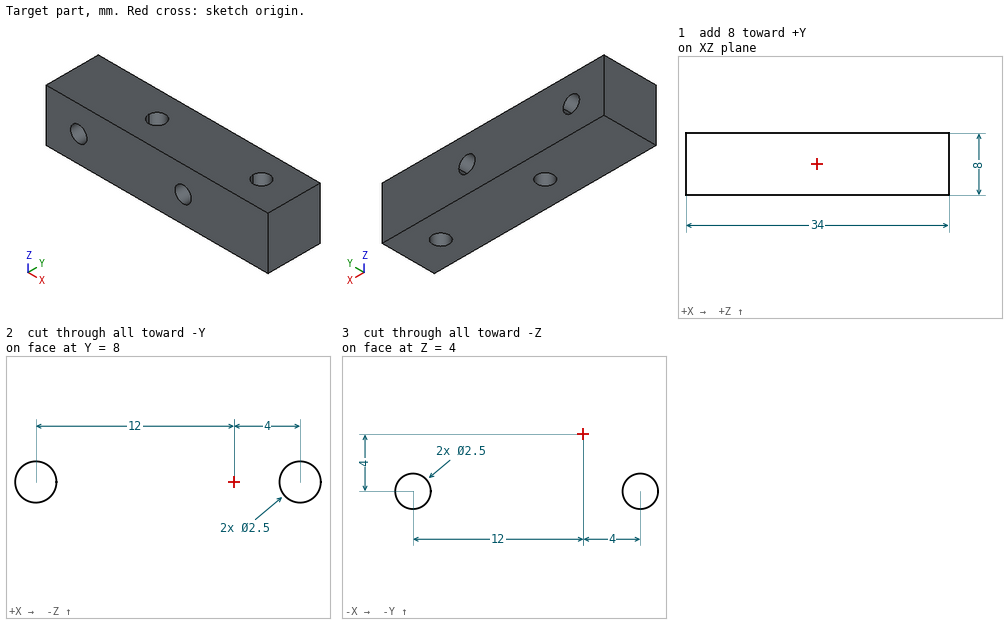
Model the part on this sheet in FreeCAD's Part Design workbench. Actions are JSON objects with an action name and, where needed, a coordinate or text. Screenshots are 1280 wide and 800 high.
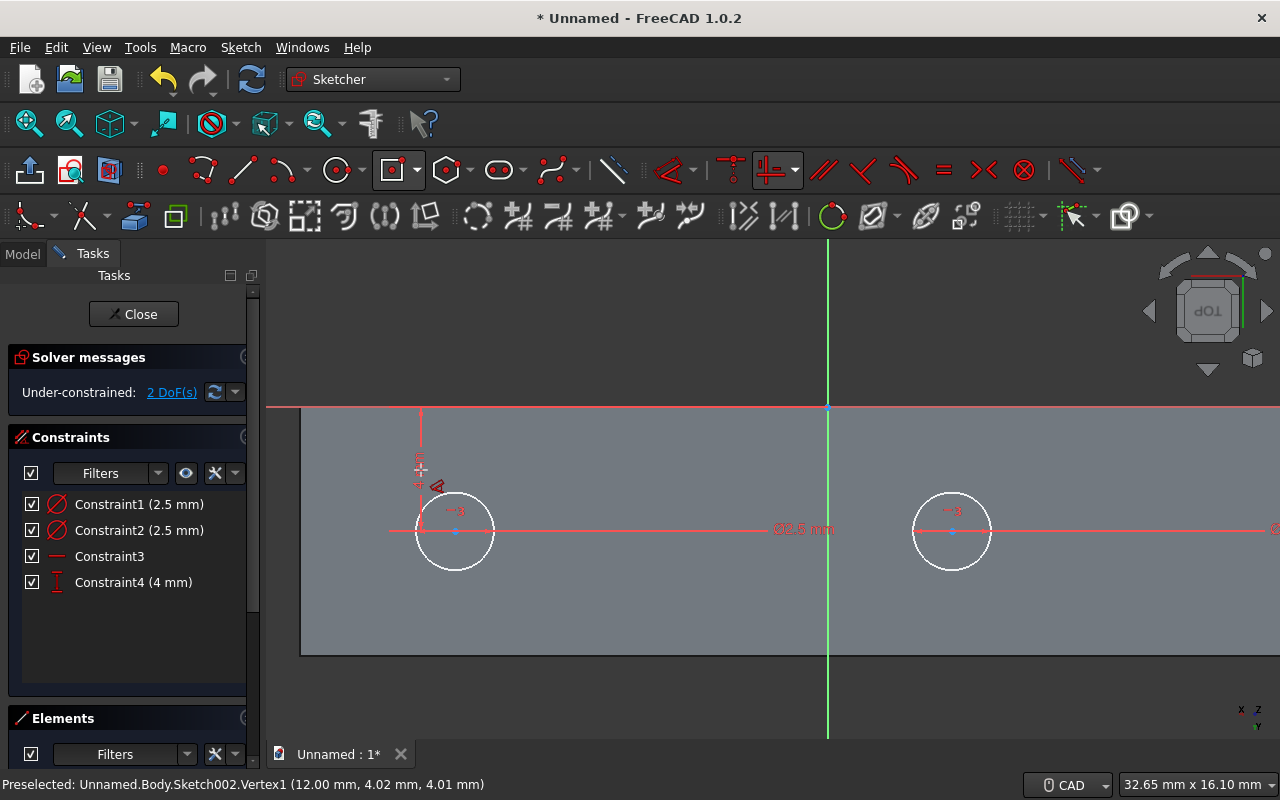
{"action": "left_click", "coordinate": [952, 531]}
{"action": "left_click", "coordinate": [890, 373]}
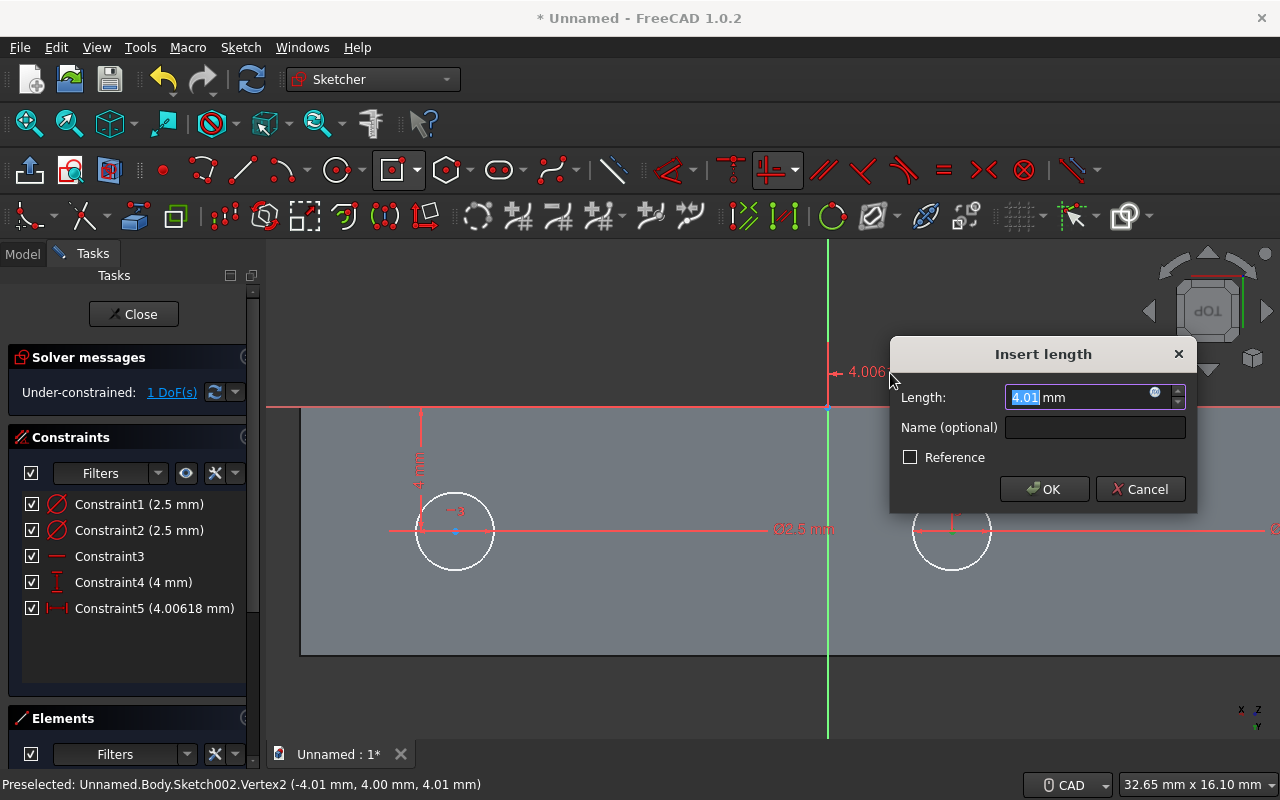
{"action": "type", "text": "4"}
{"action": "key", "text": "Return"}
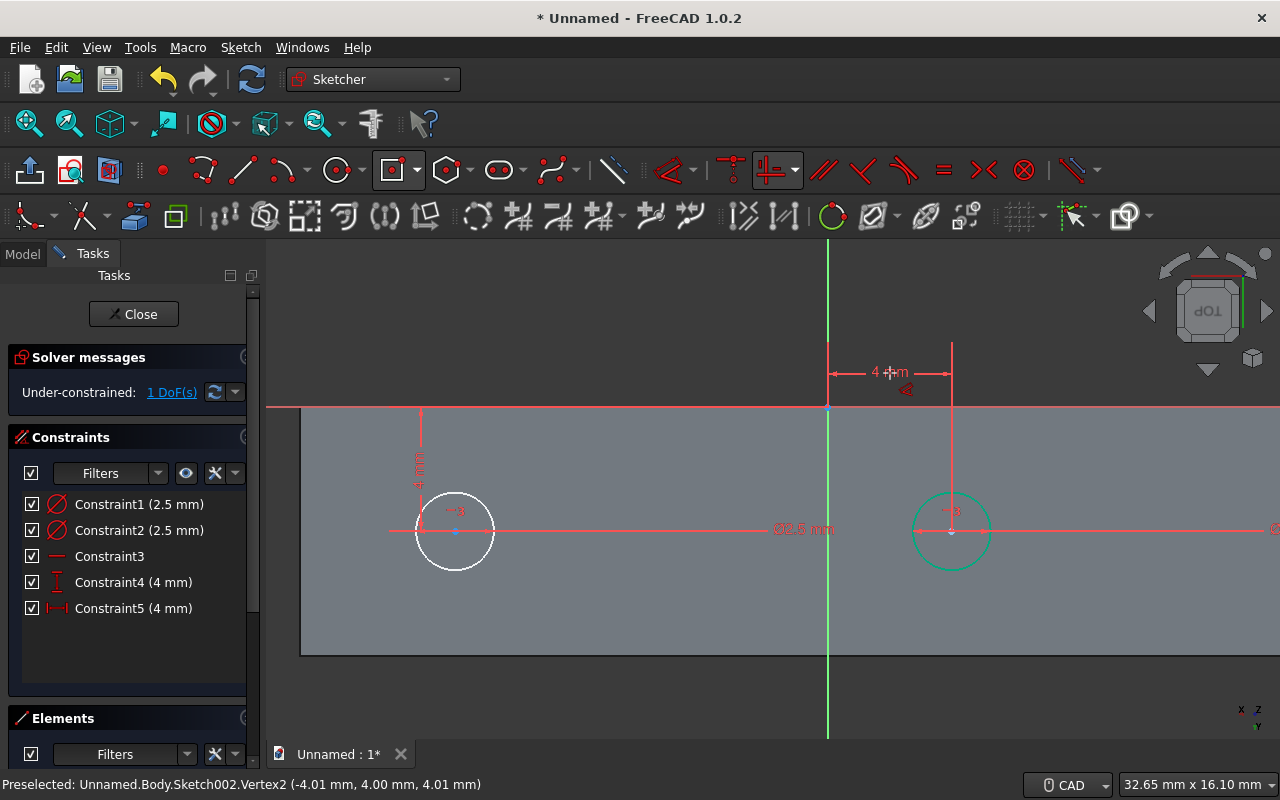
{"action": "left_click", "coordinate": [455, 531]}
{"action": "left_click", "coordinate": [641, 373]}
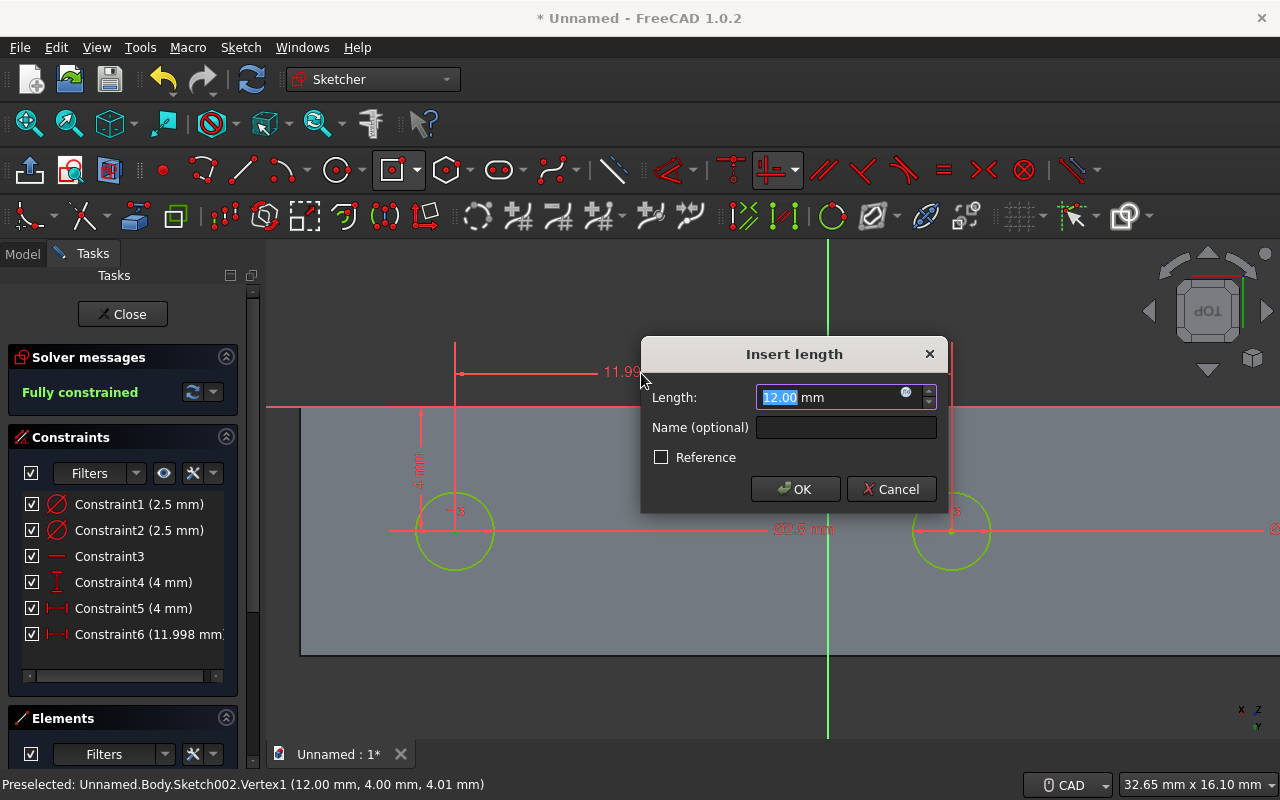
{"action": "type", "text": "12"}
{"action": "key", "text": "Return"}
{"action": "key", "text": "Escape"}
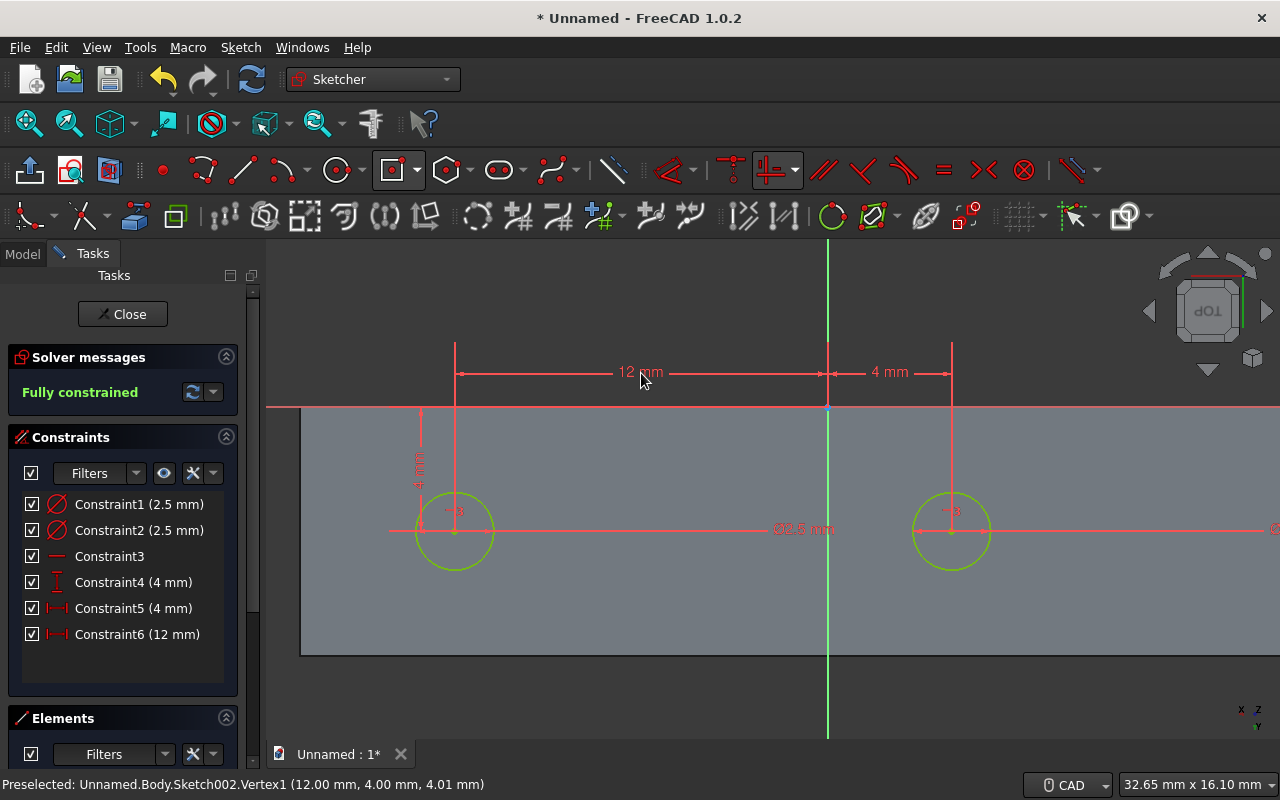
{"action": "left_click", "coordinate": [123, 314]}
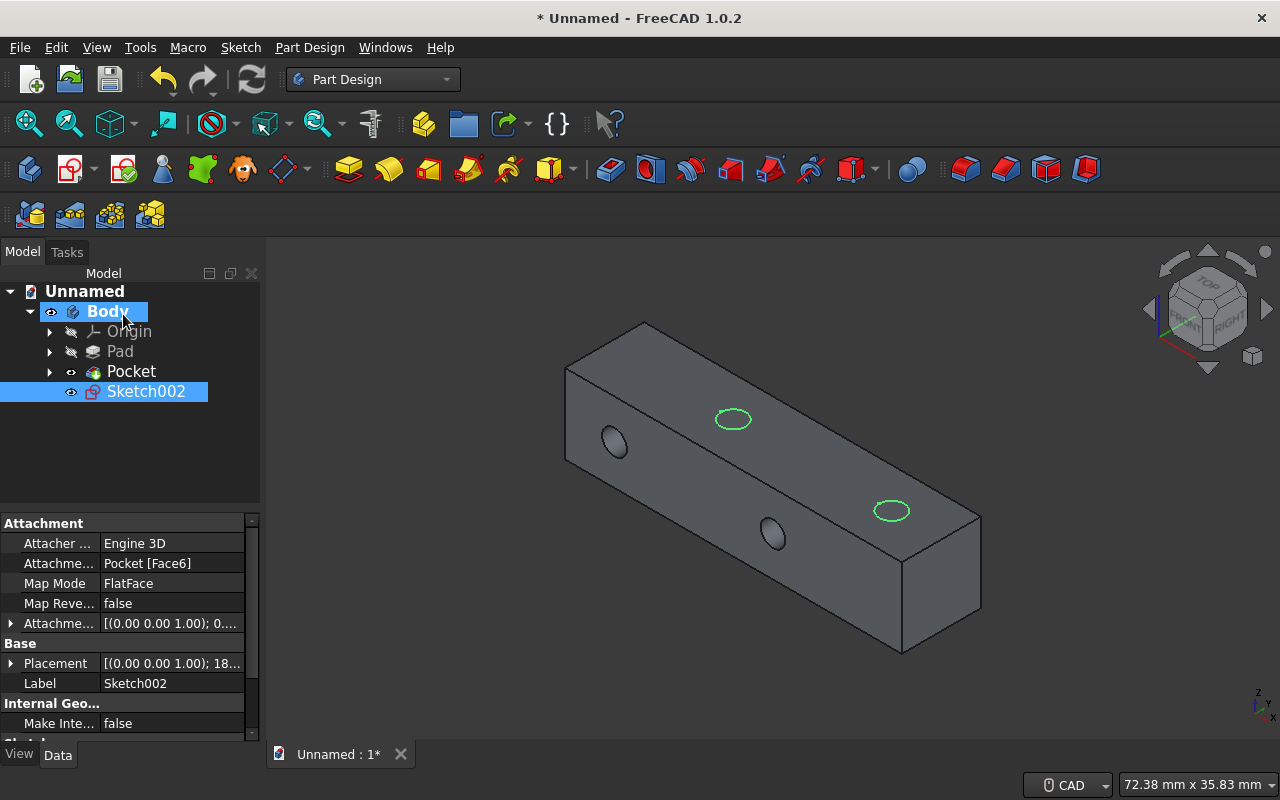
{"action": "left_click", "coordinate": [612, 170]}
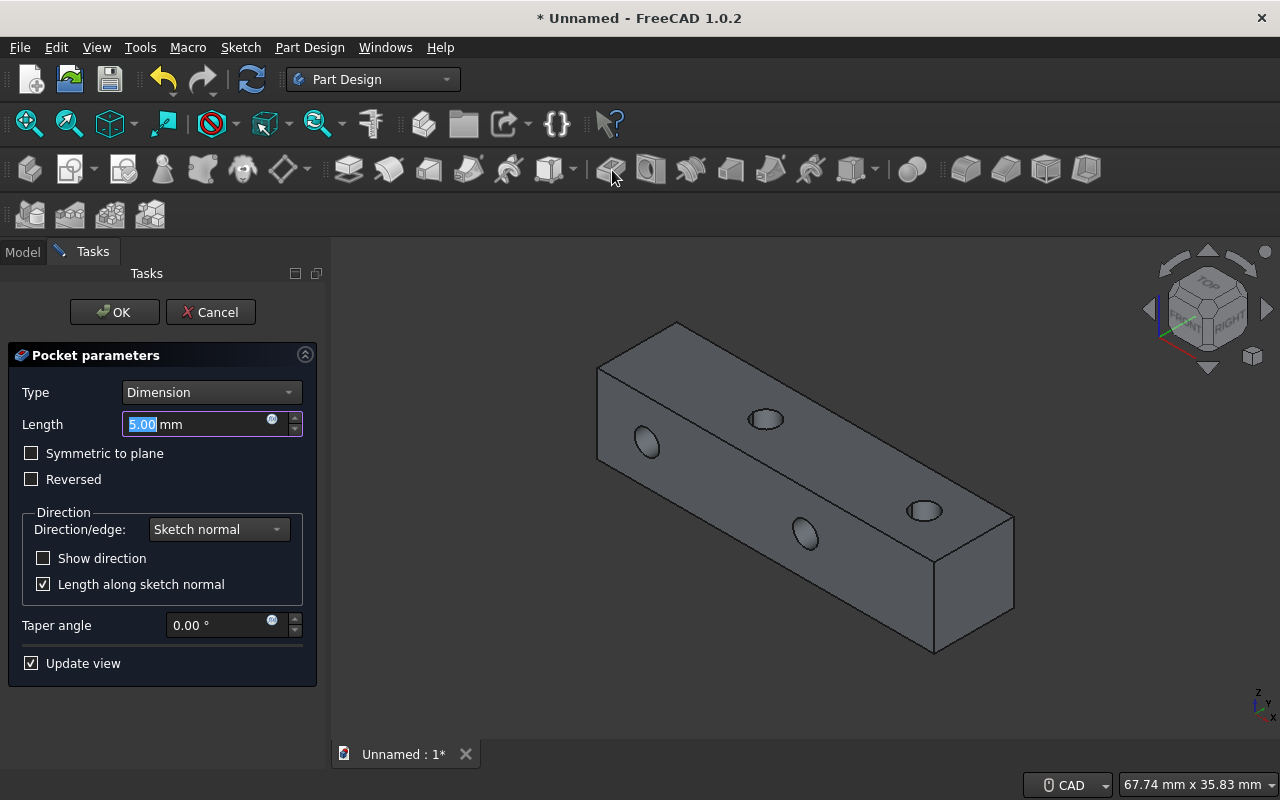
{"action": "left_click", "coordinate": [212, 392]}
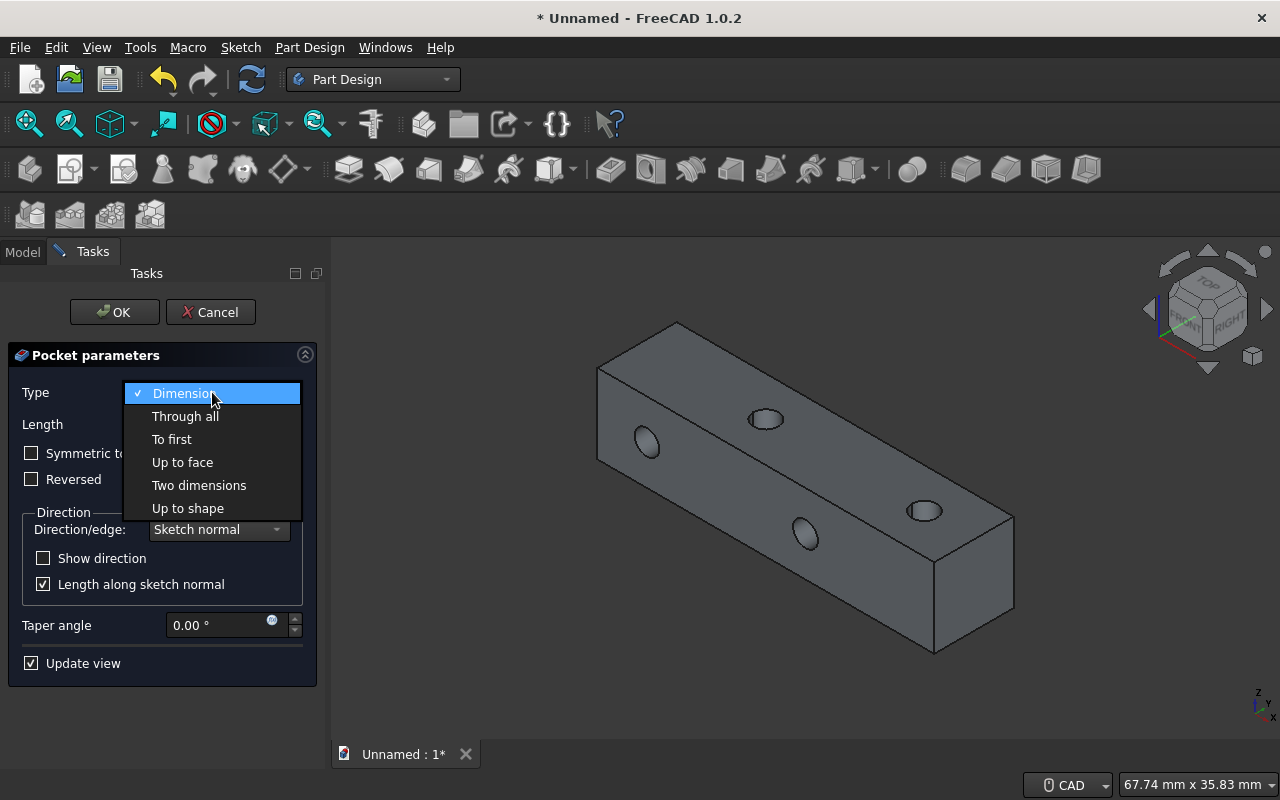
{"action": "left_click", "coordinate": [212, 416]}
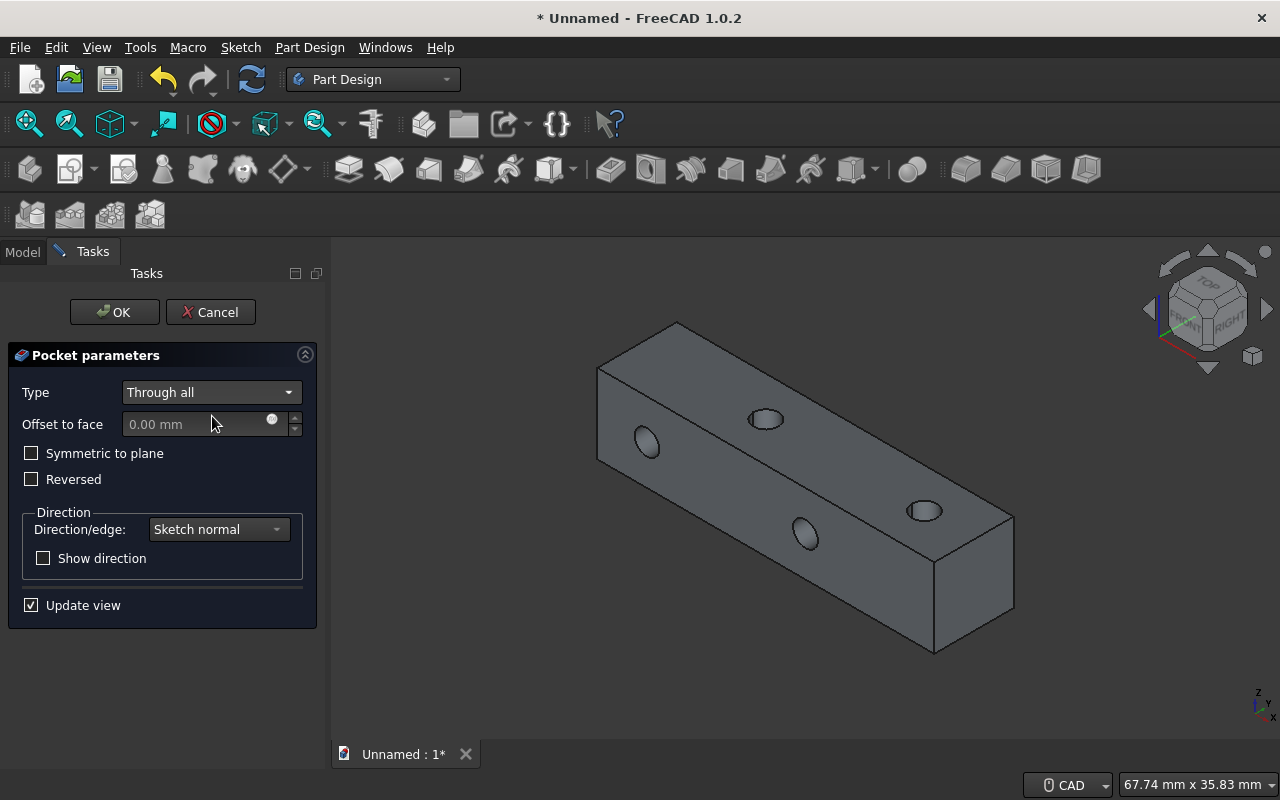
{"action": "left_click", "coordinate": [115, 312]}